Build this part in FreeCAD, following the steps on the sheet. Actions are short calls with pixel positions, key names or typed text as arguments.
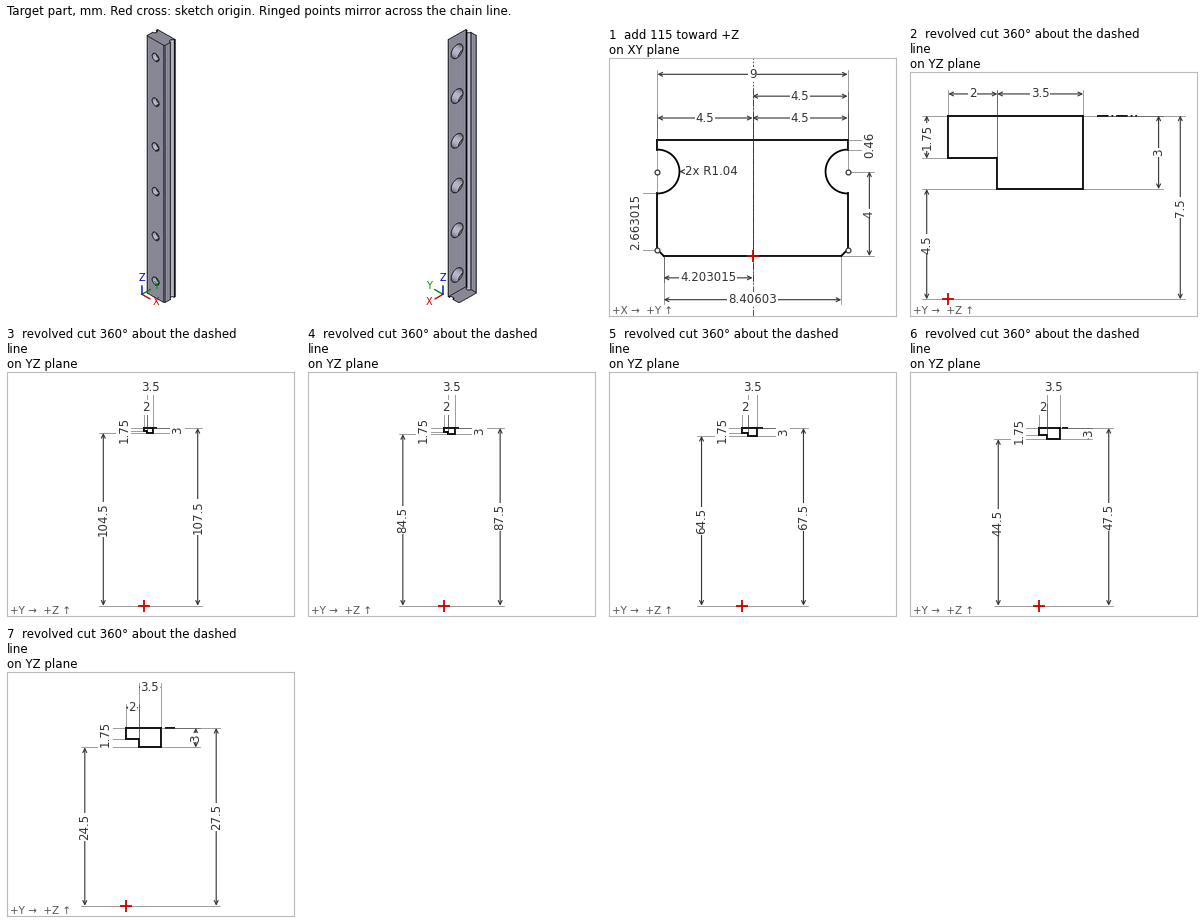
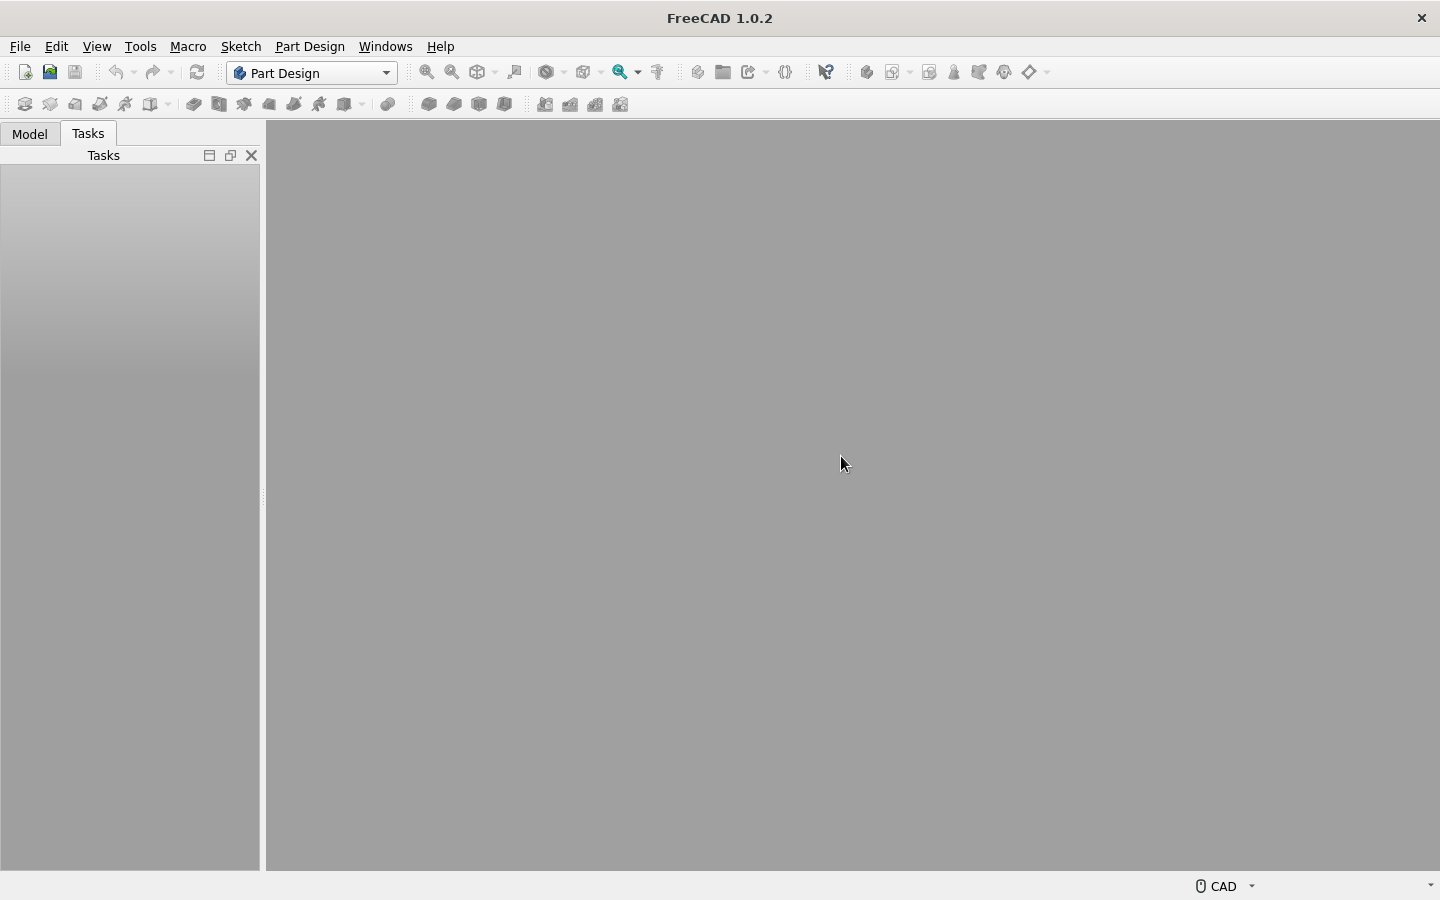
click(25, 72)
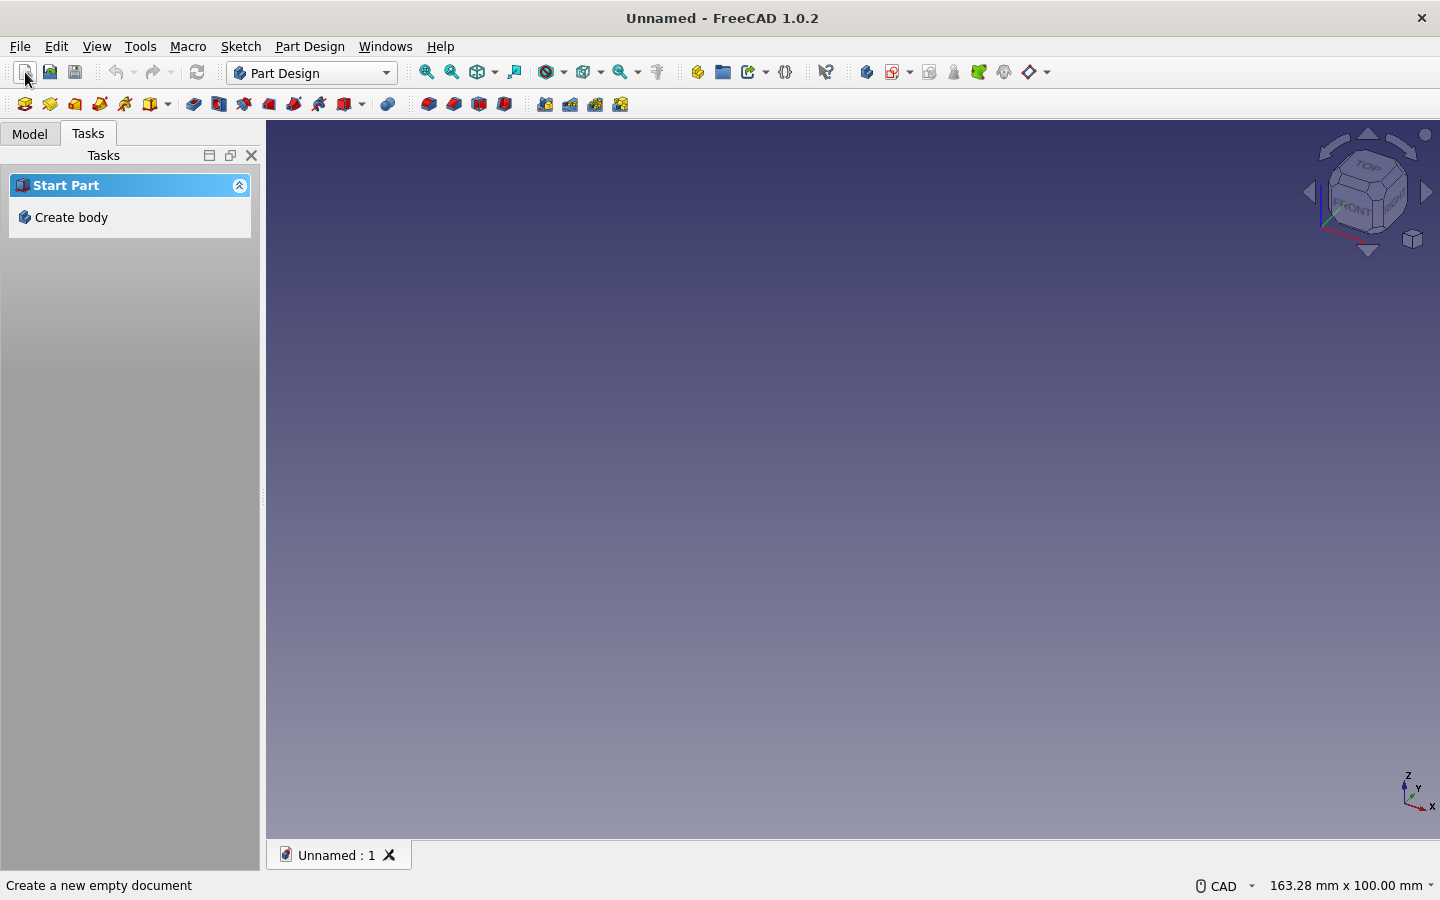
click(892, 72)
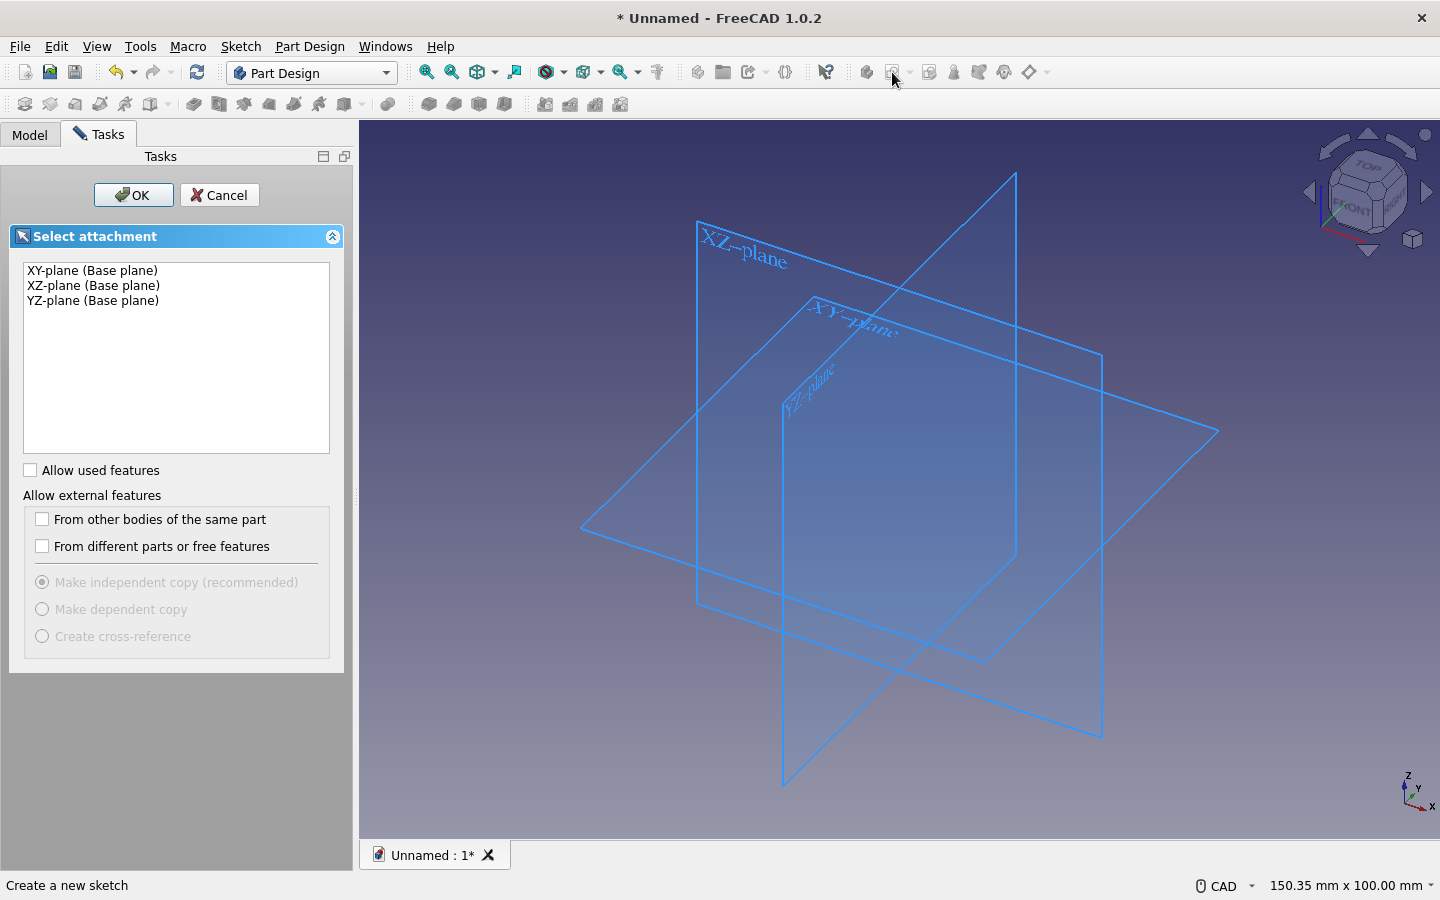
click(84, 270)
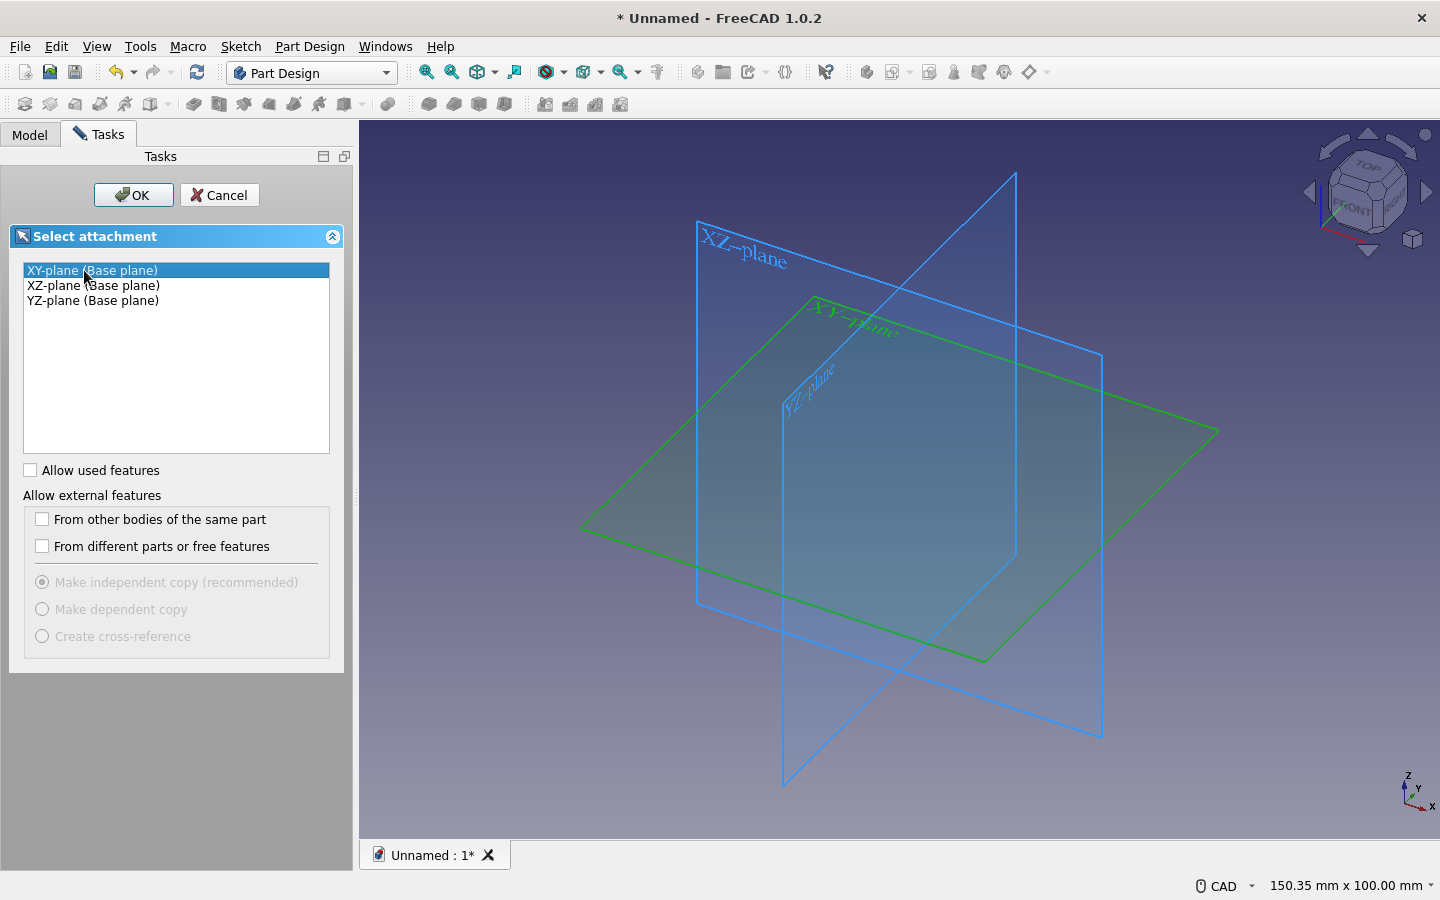
click(134, 195)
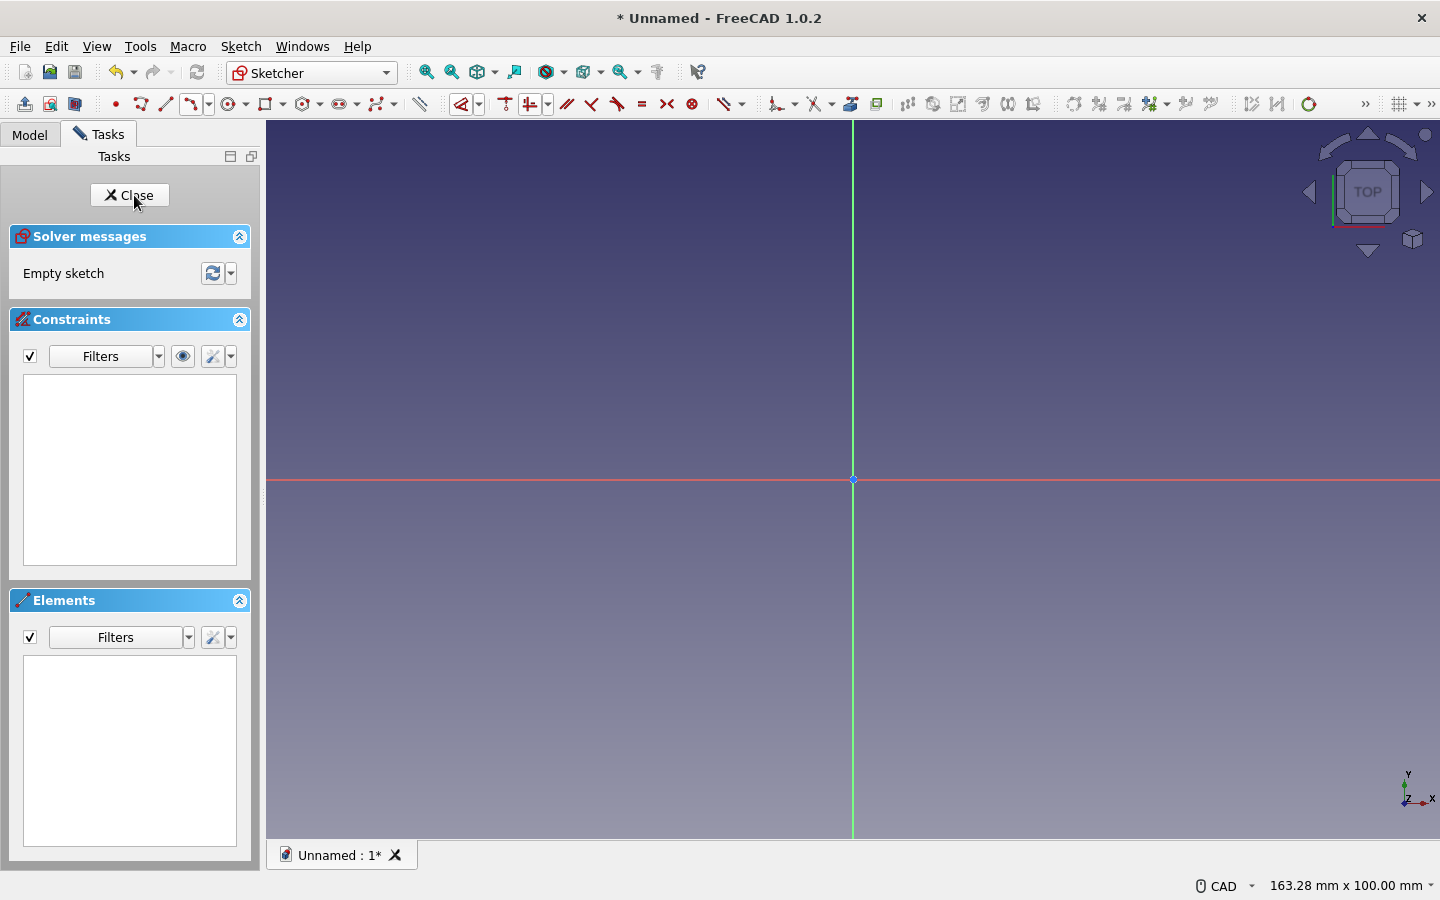
scroll(860, 458, up, 12)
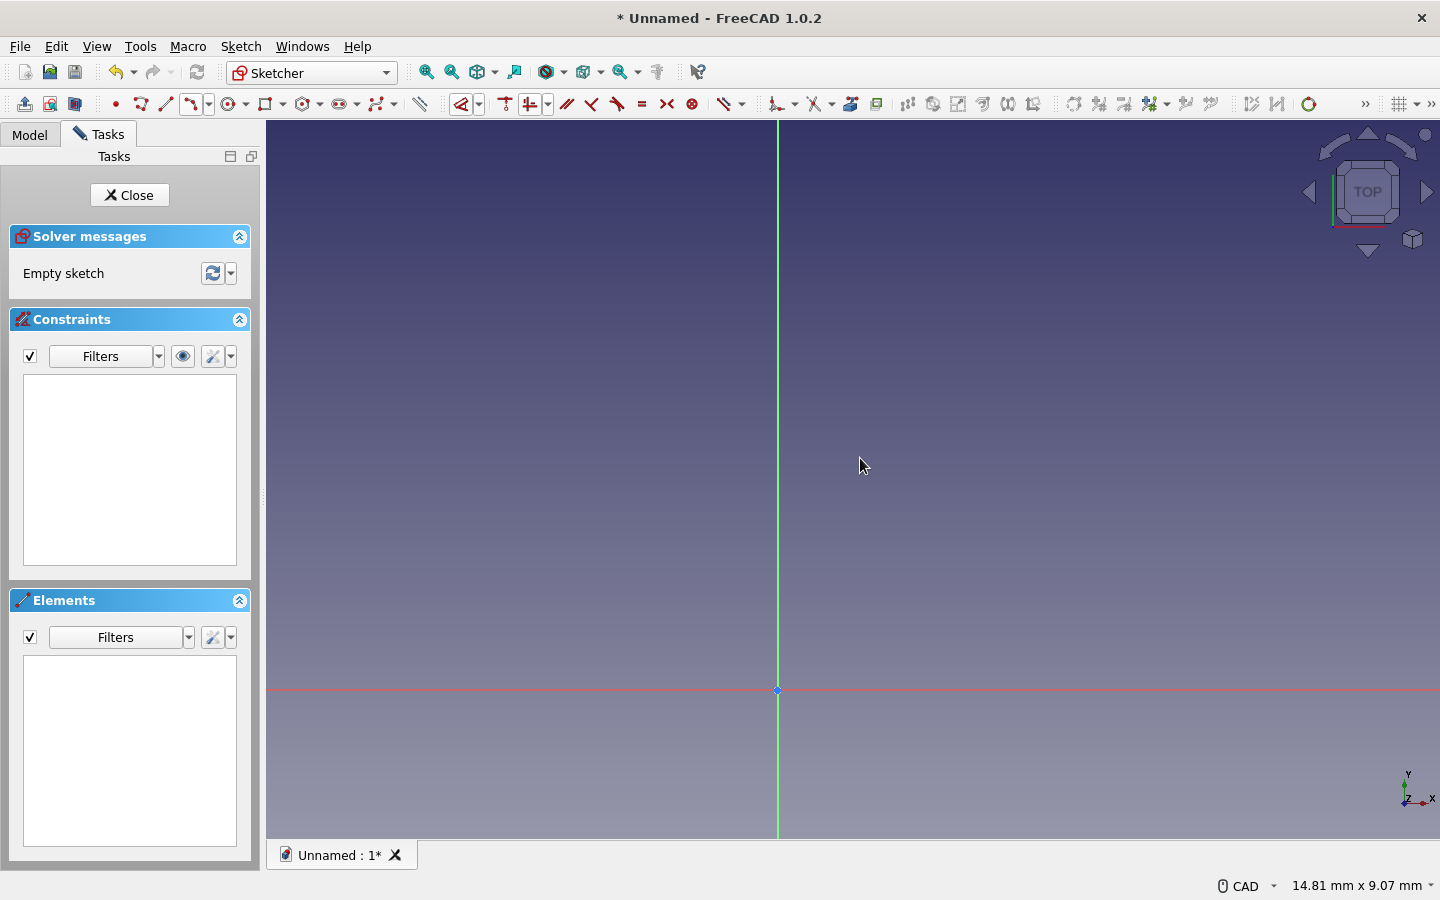
key(g)
key(m)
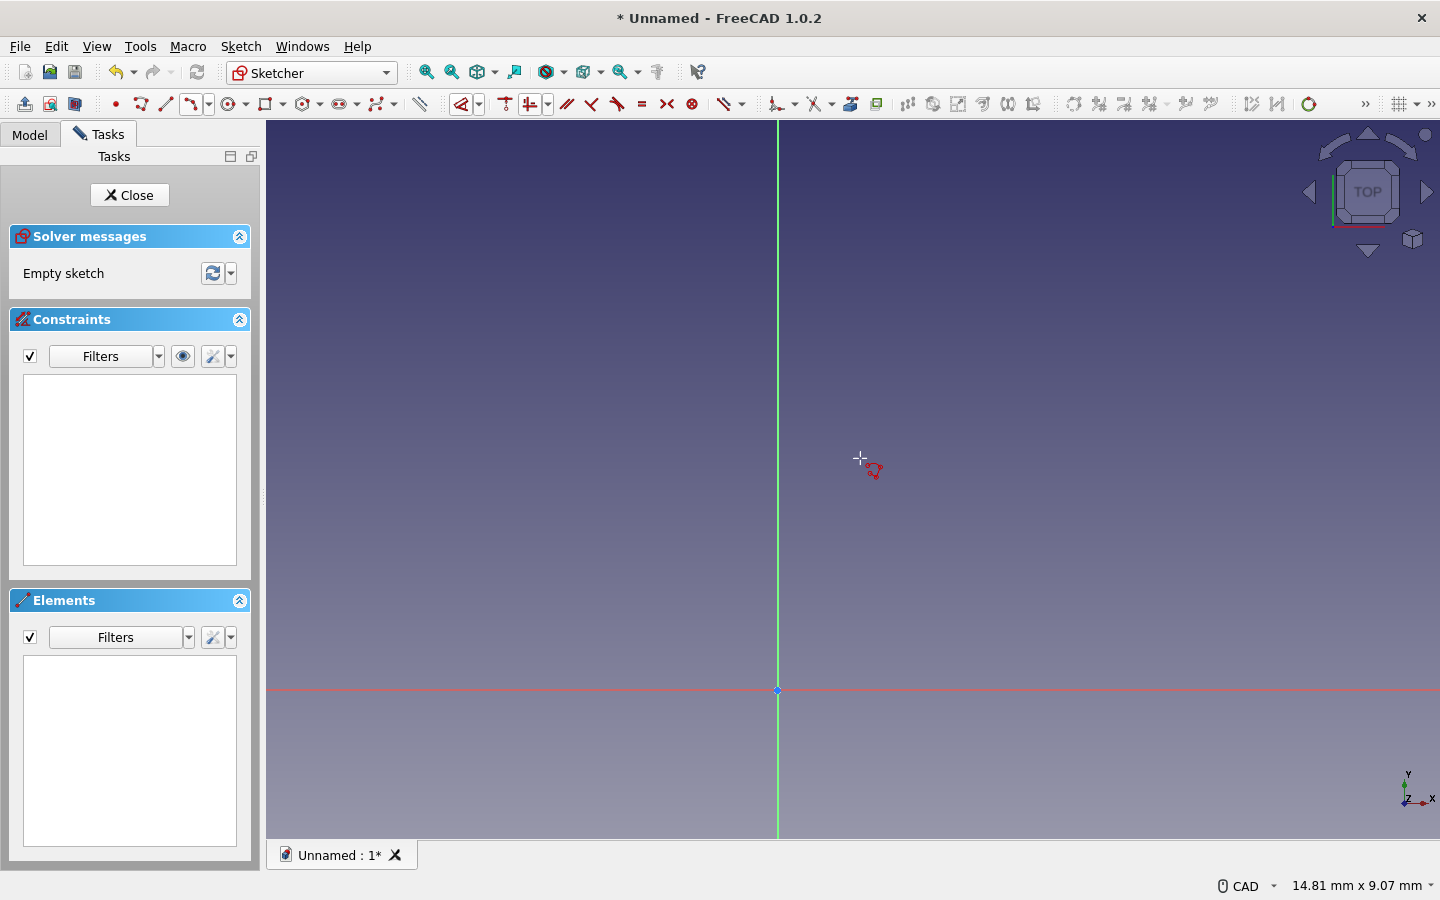
click(421, 456)
click(421, 667)
click(445, 690)
click(1111, 681)
click(1134, 667)
click(1134, 456)
right_click(1134, 456)